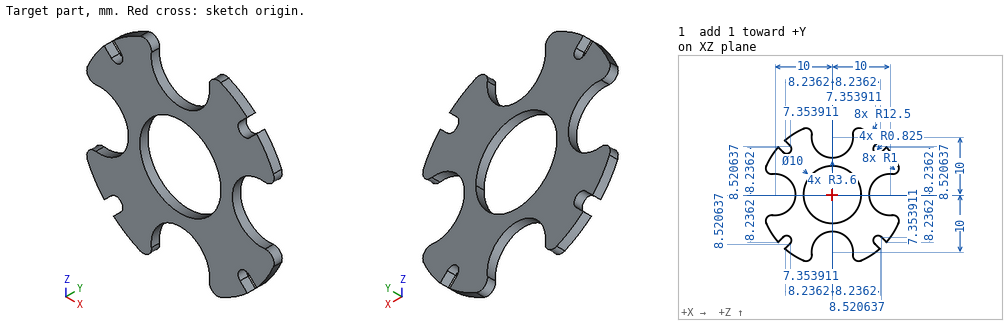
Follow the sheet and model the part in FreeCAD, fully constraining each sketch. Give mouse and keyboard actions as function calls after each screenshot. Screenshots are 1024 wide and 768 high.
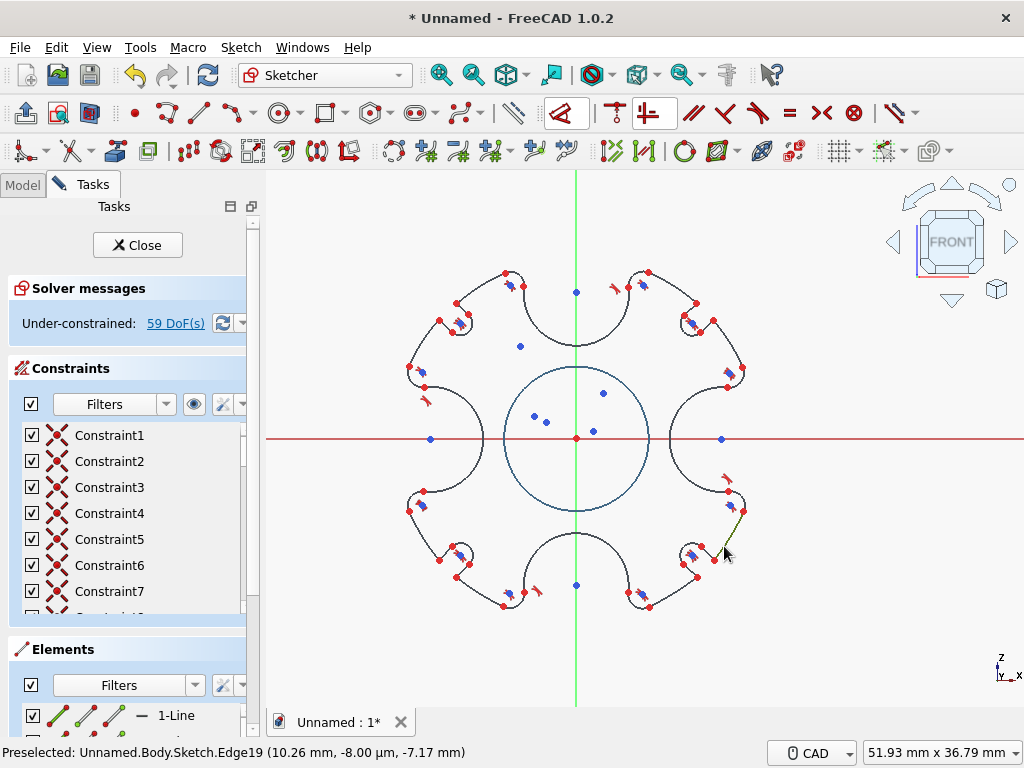
click(616, 114)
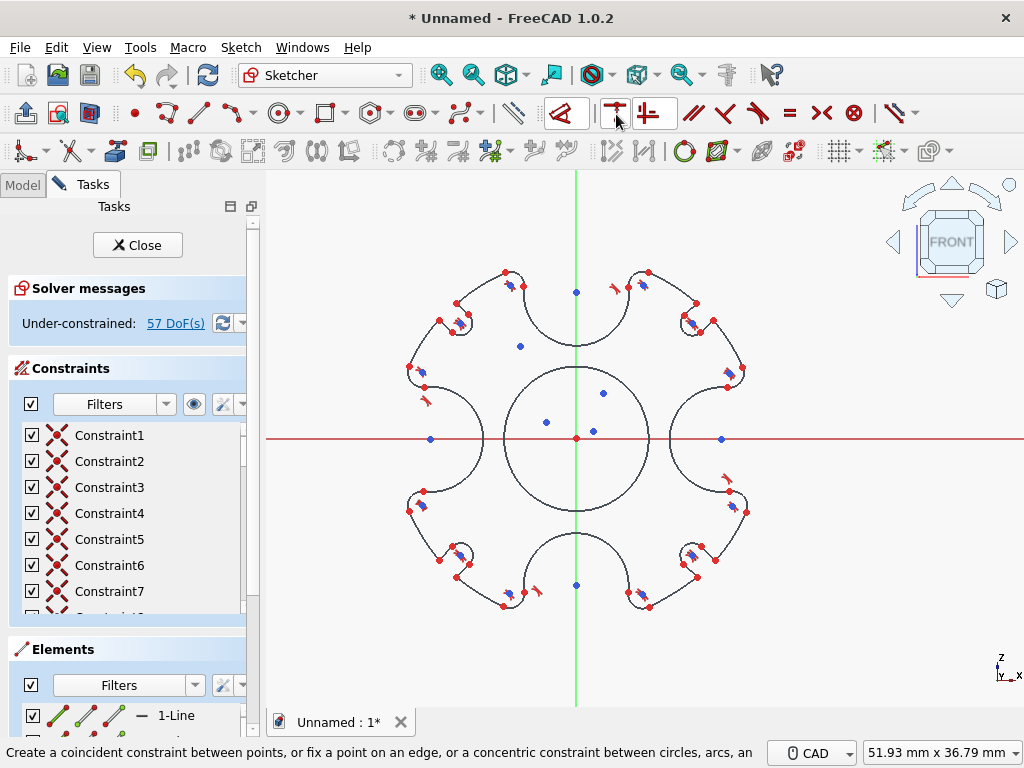
click(627, 387)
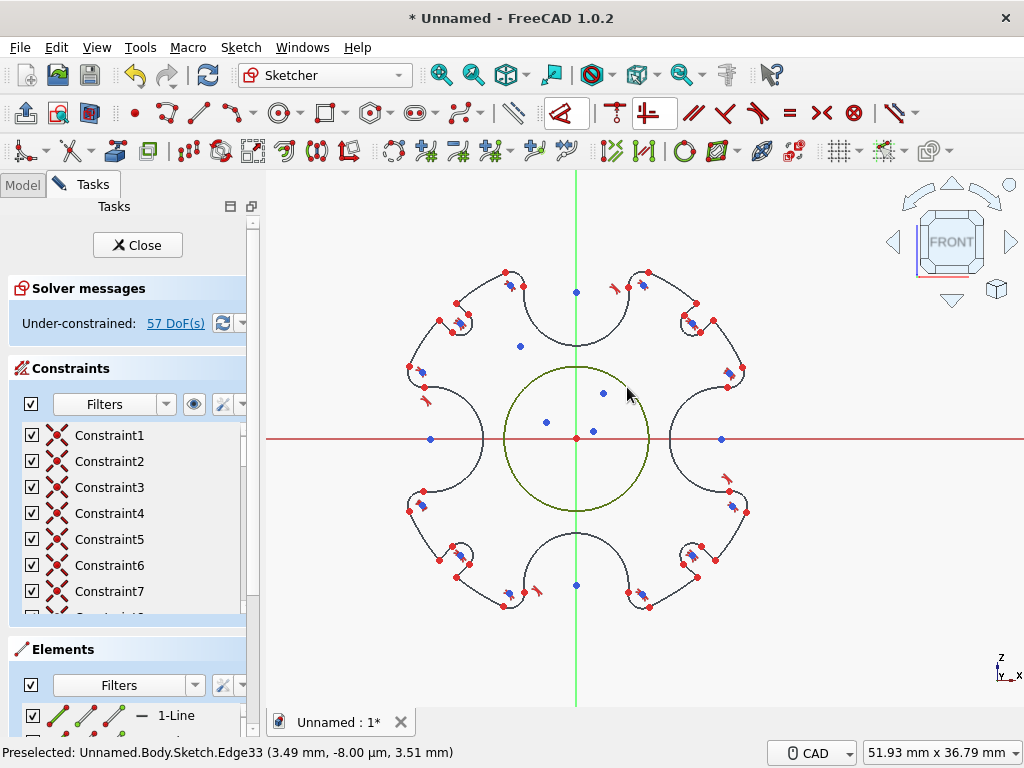
click(664, 599)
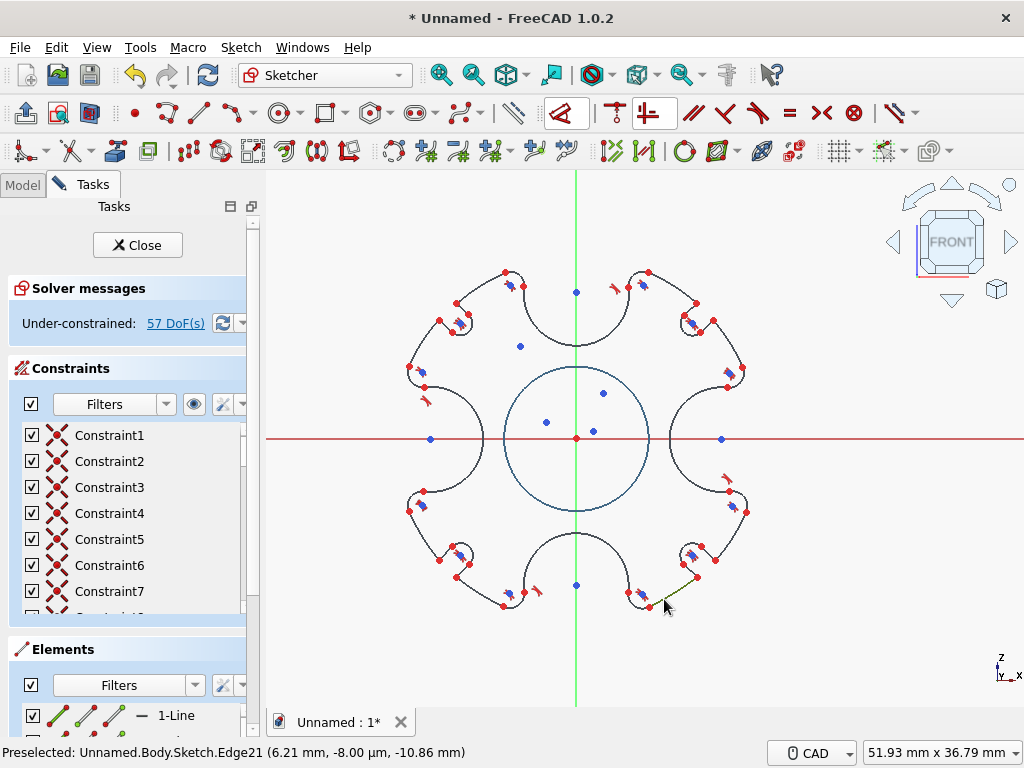
click(616, 114)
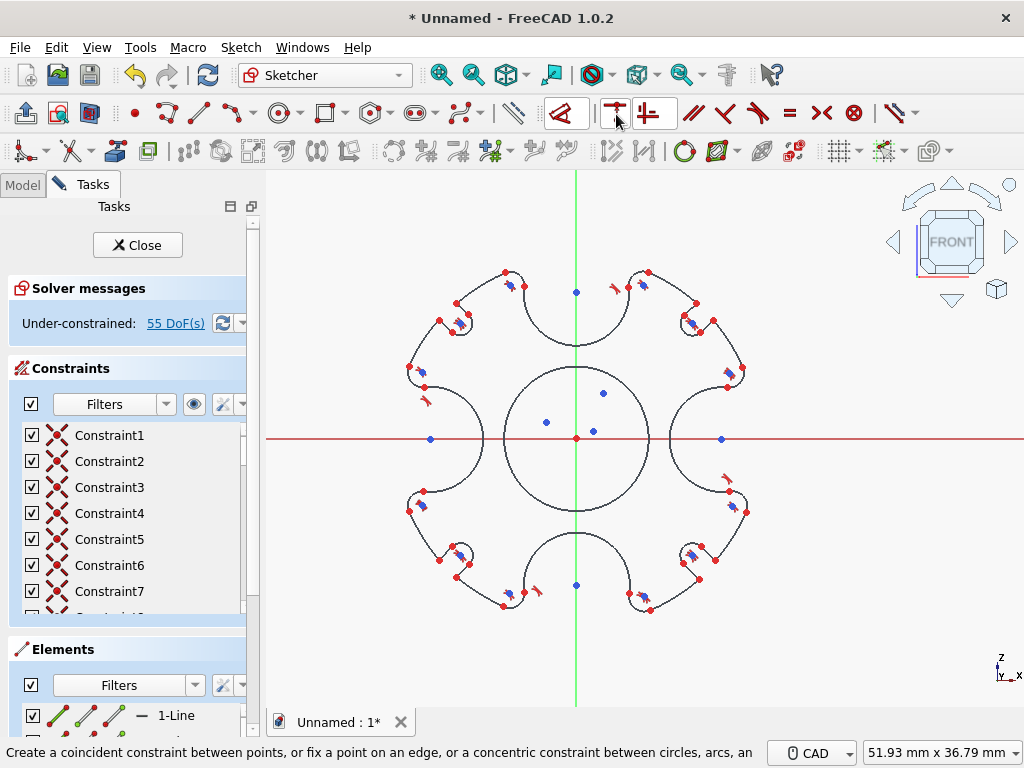
click(627, 387)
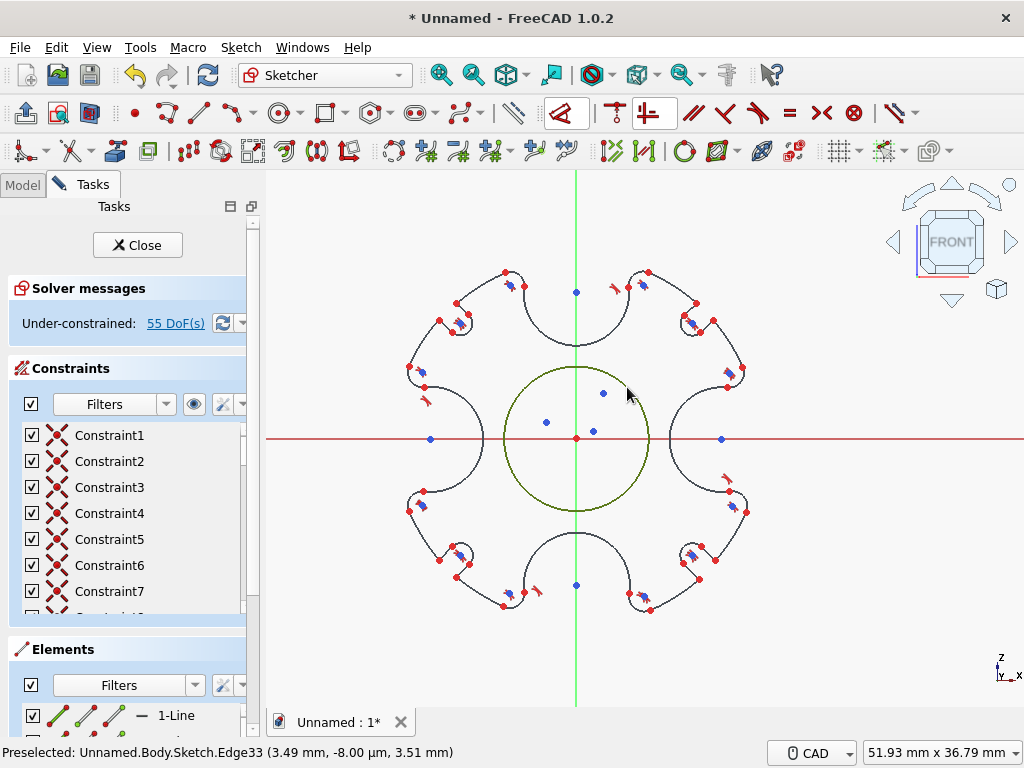
click(470, 587)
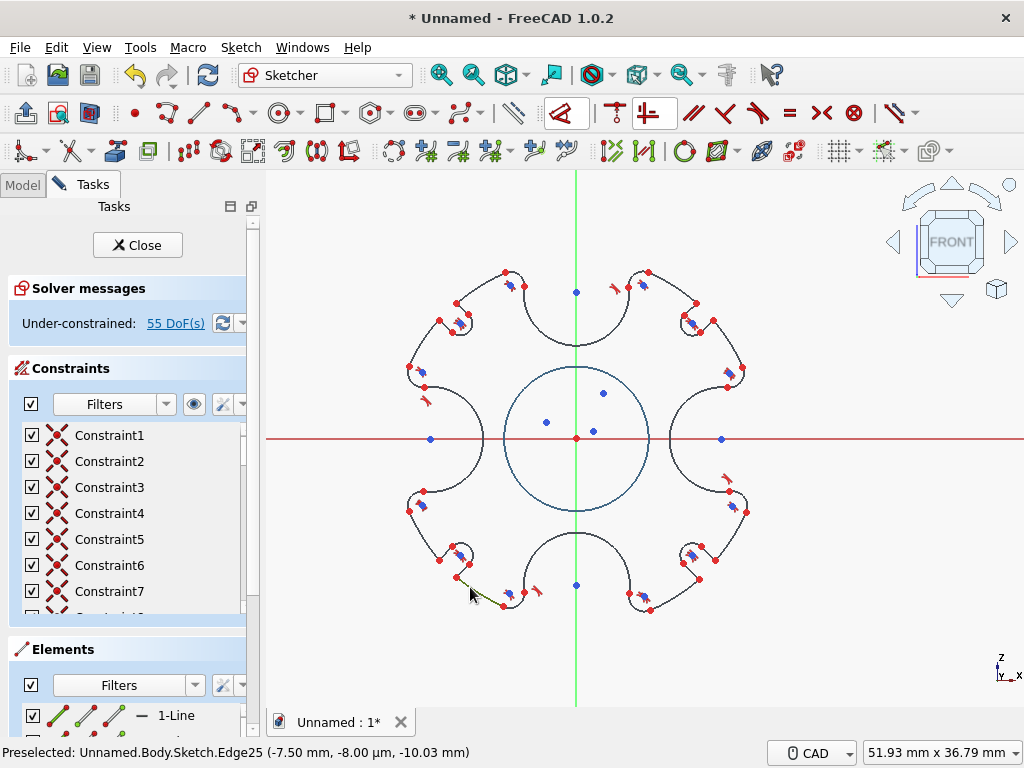
click(616, 114)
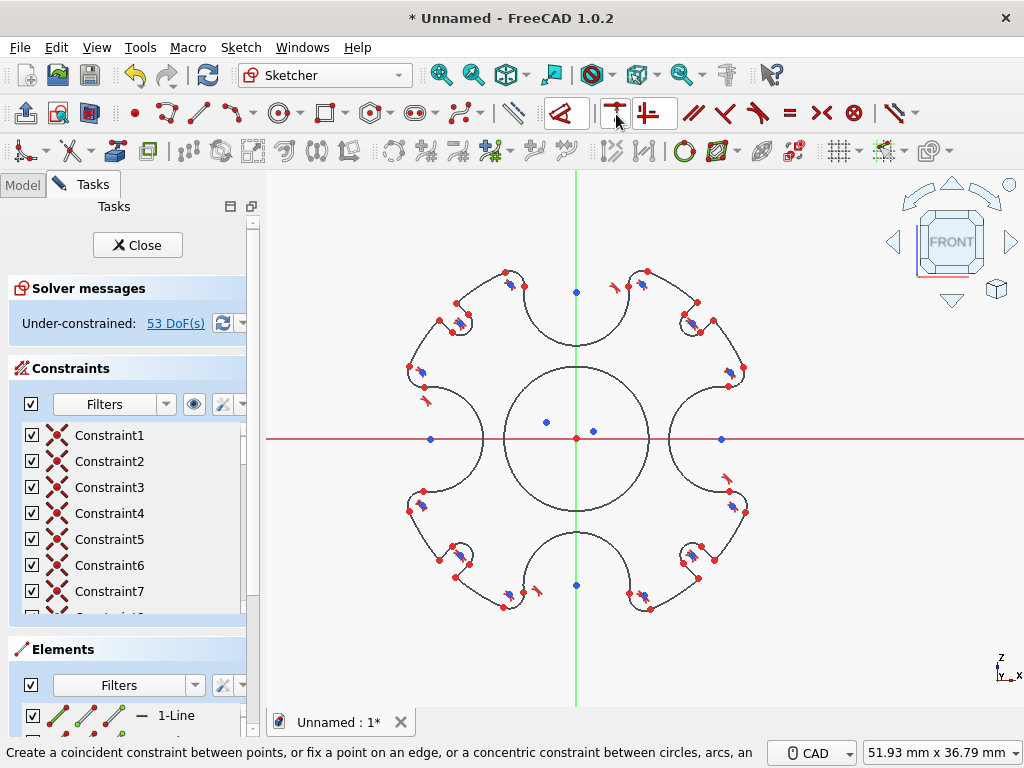
click(627, 387)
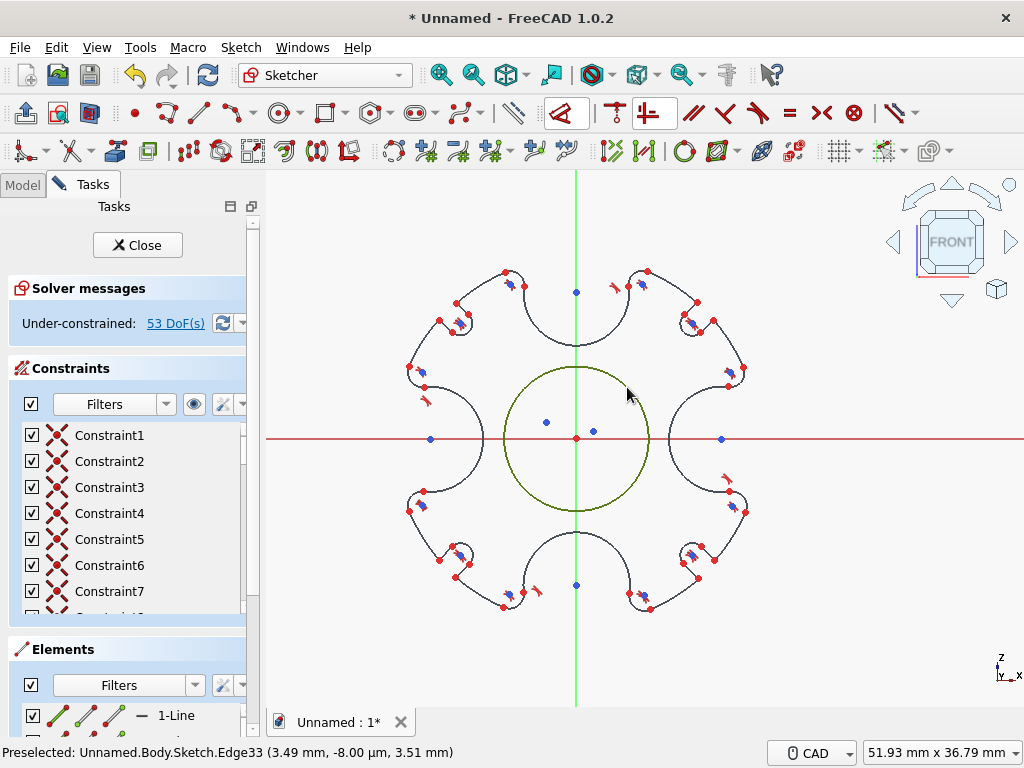
click(417, 527)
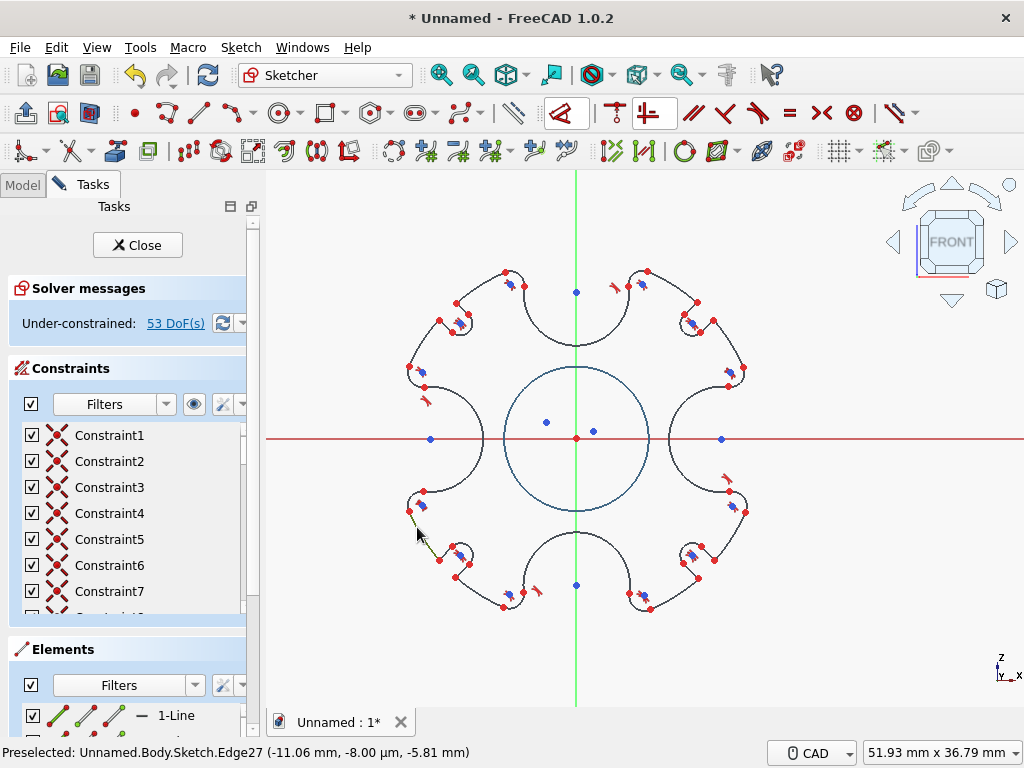
click(616, 114)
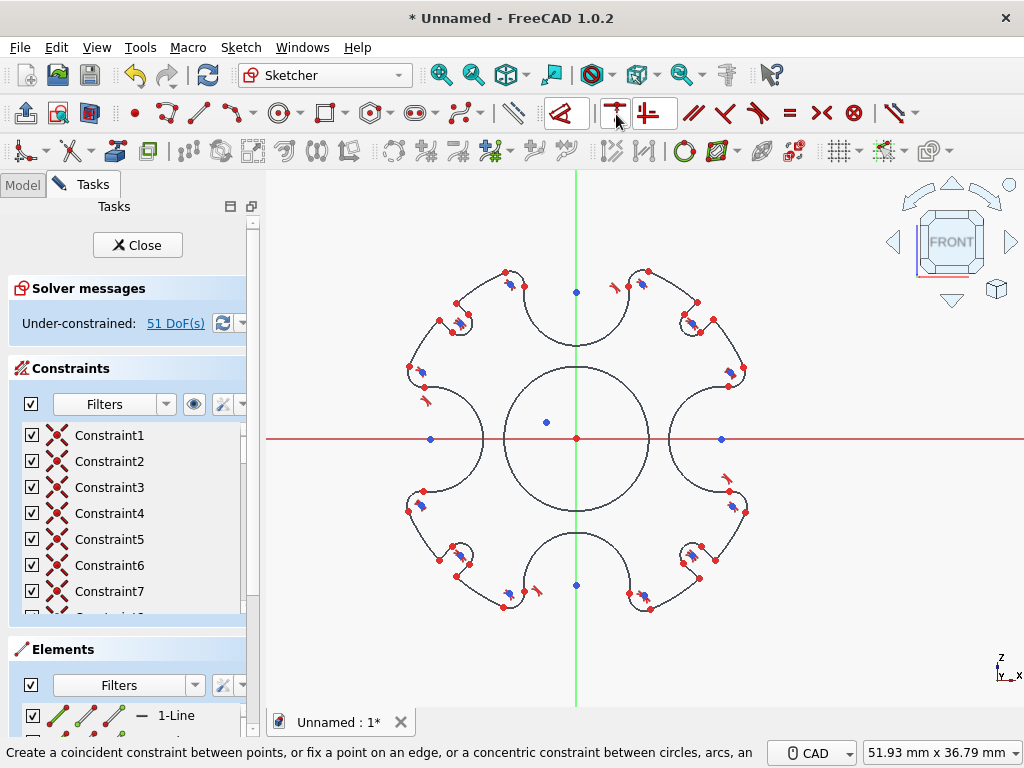
click(627, 387)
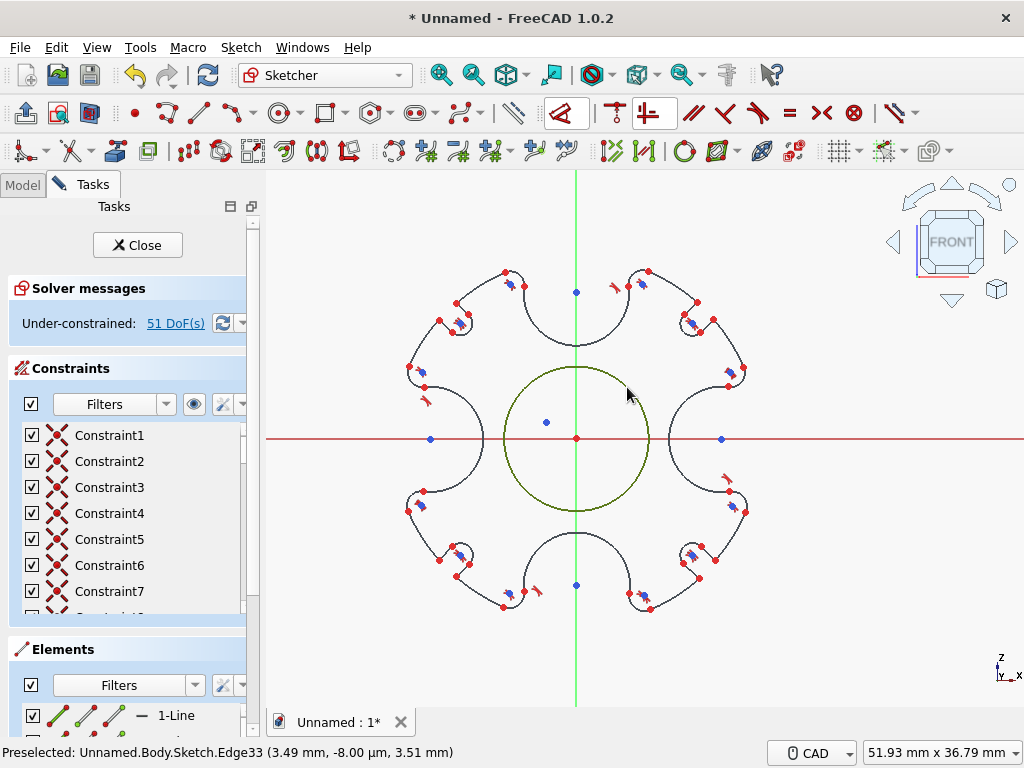
click(428, 333)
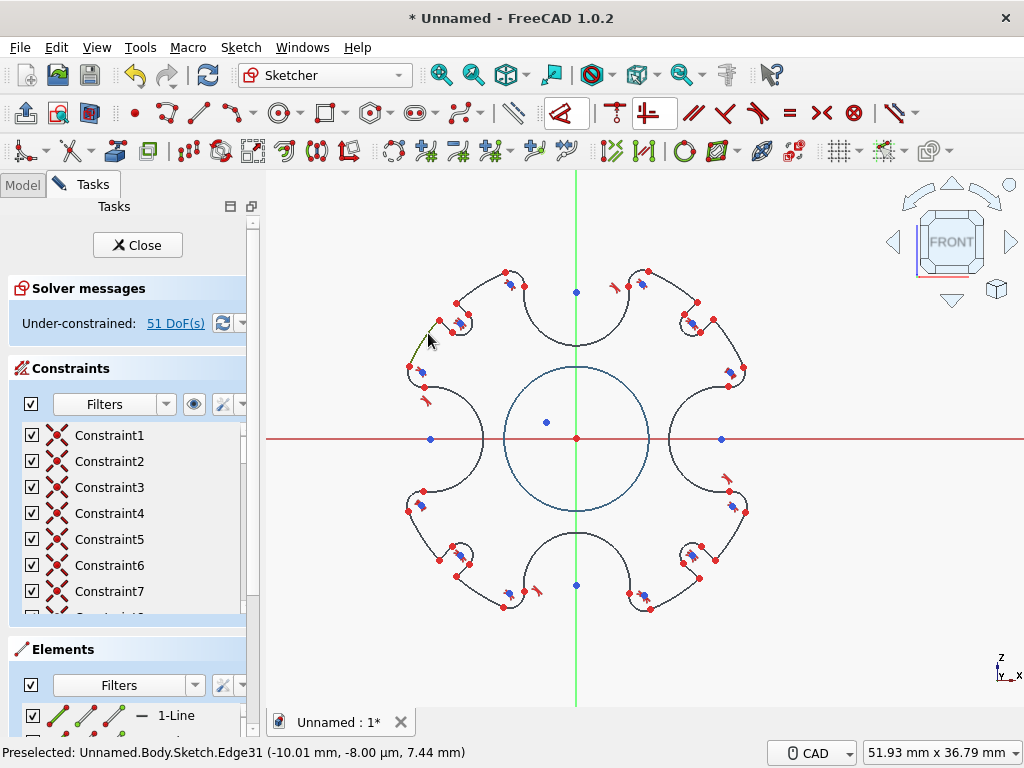
click(616, 114)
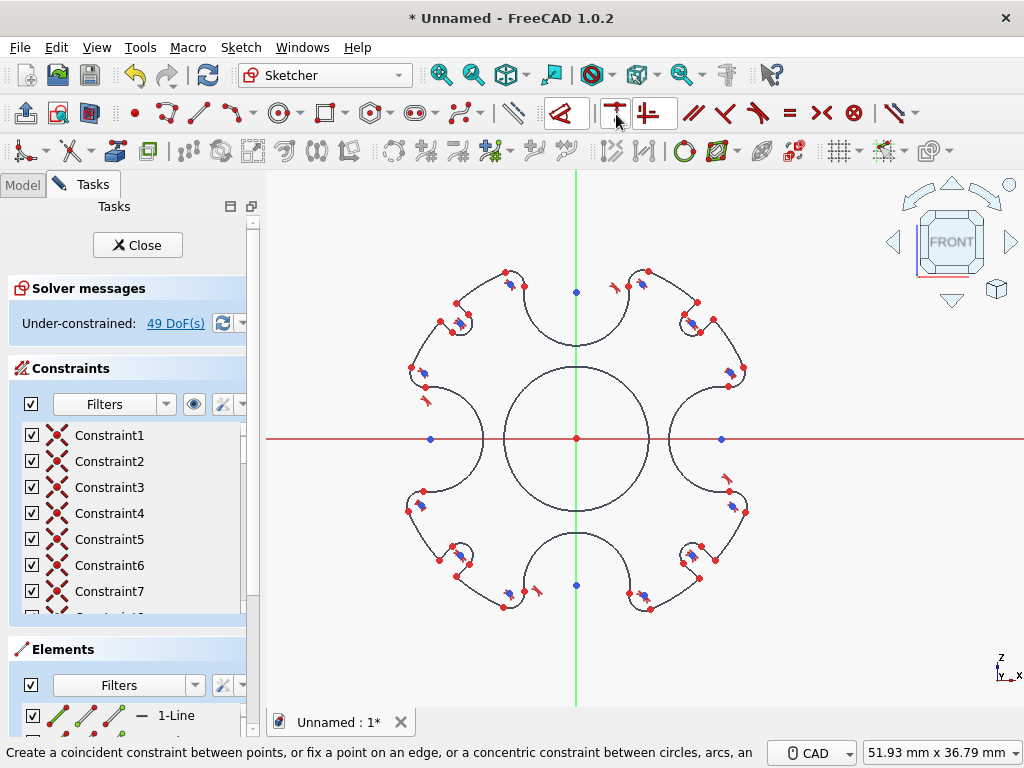
click(519, 274)